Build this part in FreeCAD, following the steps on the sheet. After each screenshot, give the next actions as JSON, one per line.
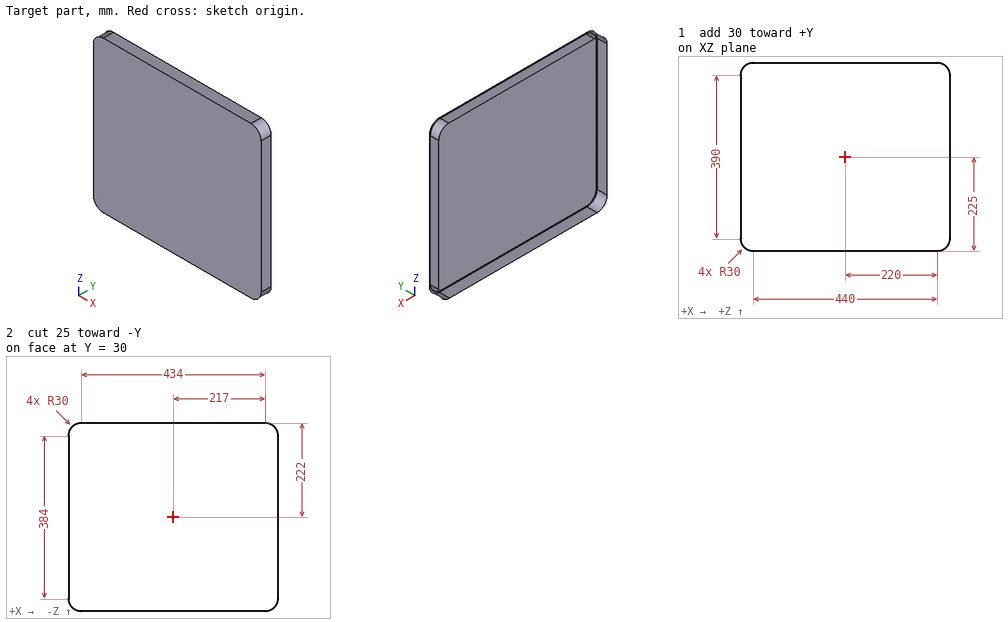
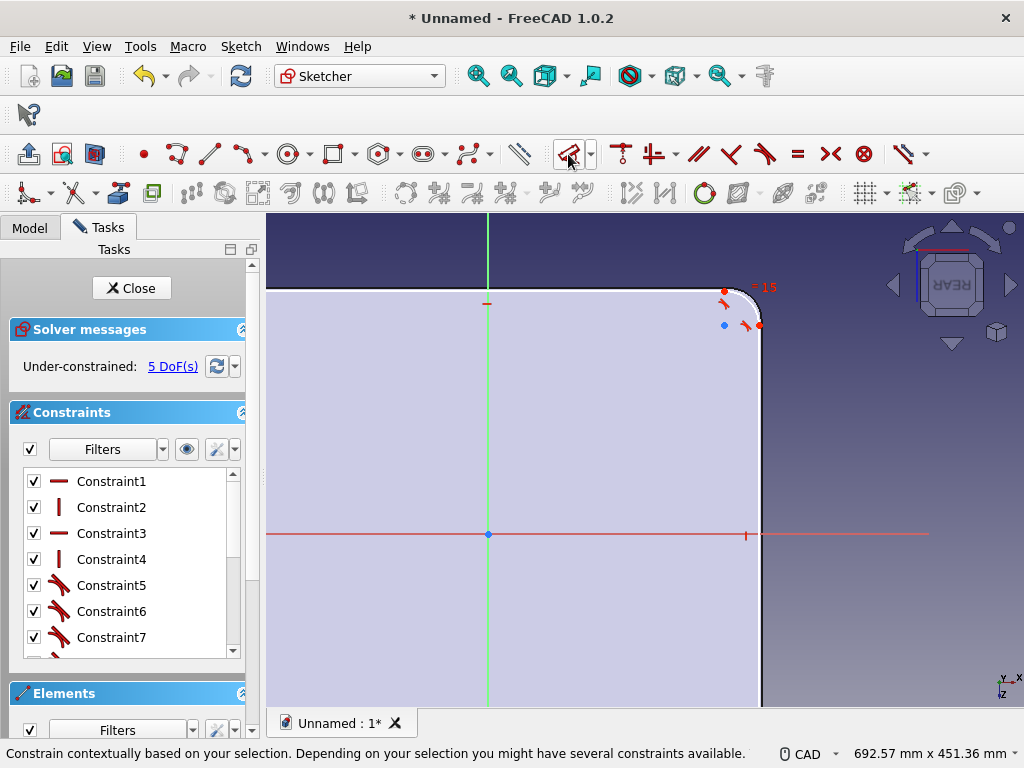
{"action": "scroll", "coordinate": [756, 309], "scroll_direction": "down", "scroll_amount": 2}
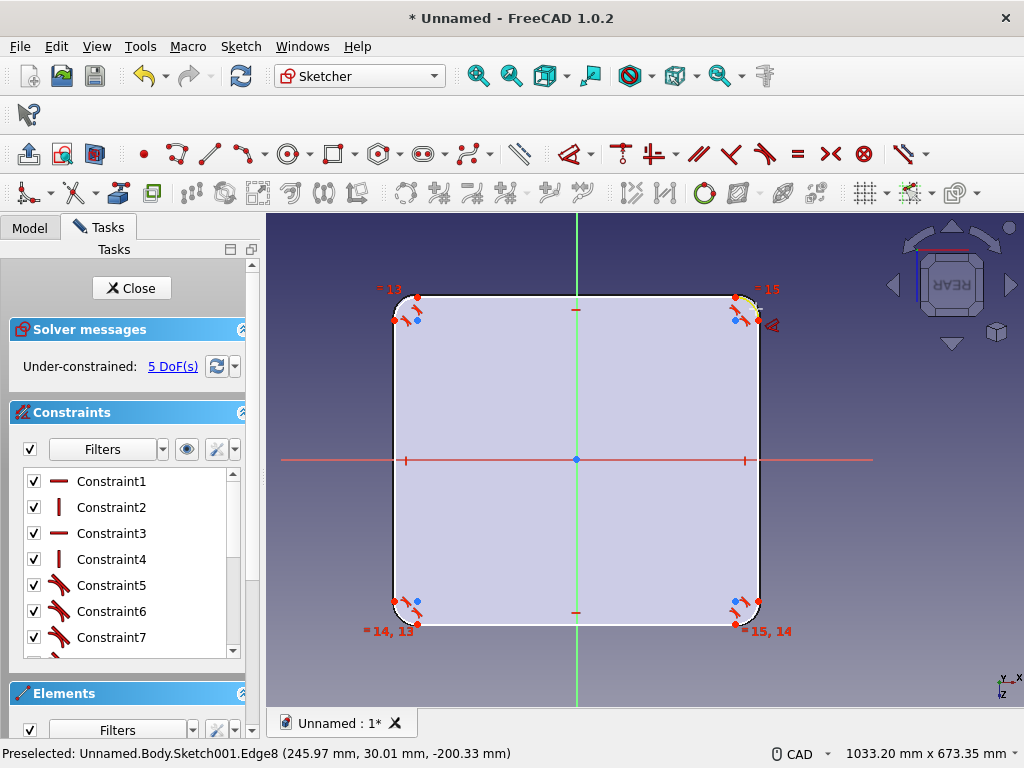
{"action": "scroll", "coordinate": [407, 300], "scroll_direction": "up", "scroll_amount": 3}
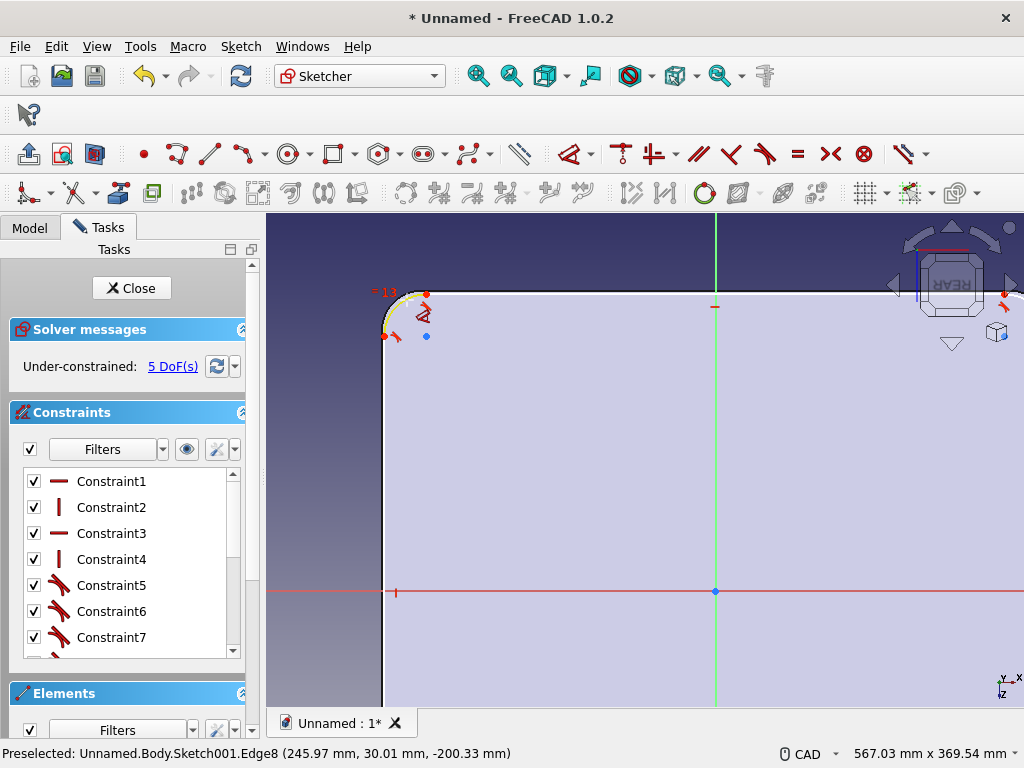
{"action": "left_click", "coordinate": [407, 299]}
{"action": "left_click", "coordinate": [392, 271]}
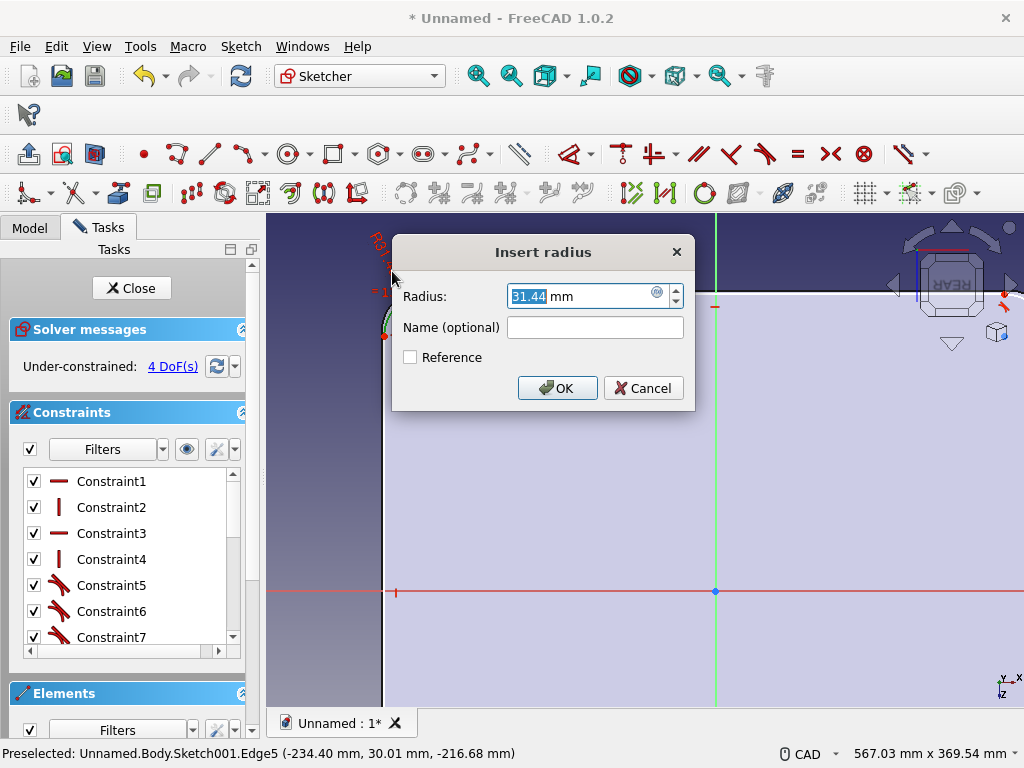
{"action": "type", "text": "30"}
{"action": "key", "text": "Return"}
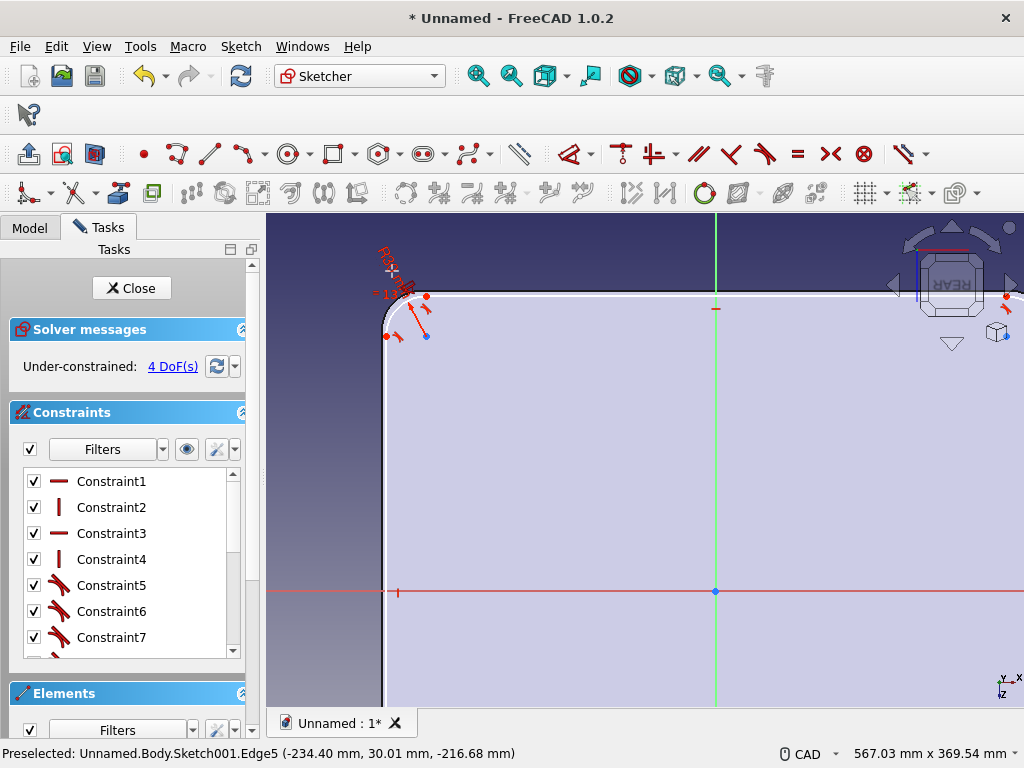
{"action": "left_click", "coordinate": [832, 296]}
{"action": "left_click", "coordinate": [643, 262]}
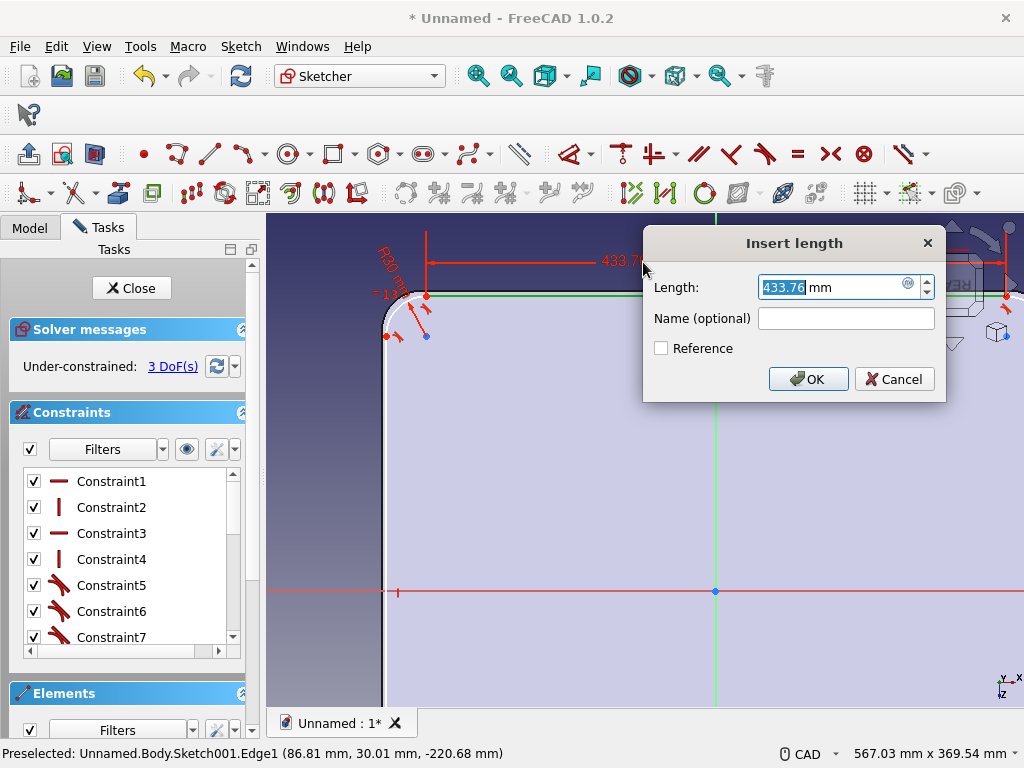
{"action": "type", "text": "434"}
{"action": "key", "text": "Return"}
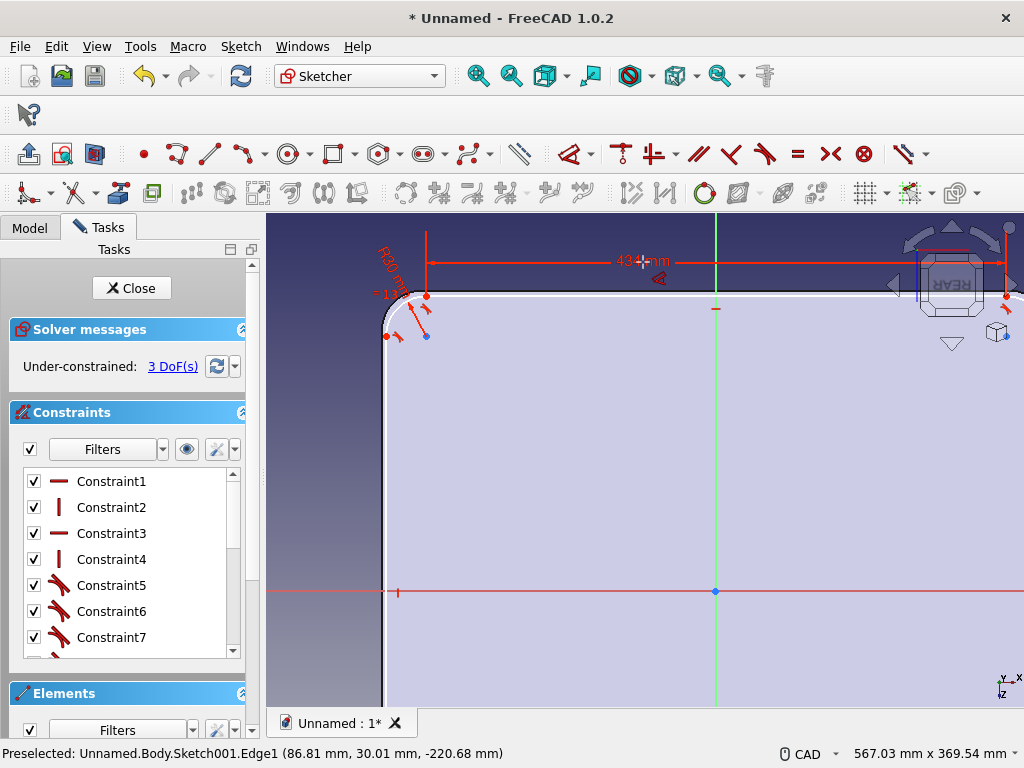
{"action": "left_click", "coordinate": [386, 490]}
{"action": "left_click", "coordinate": [352, 508]}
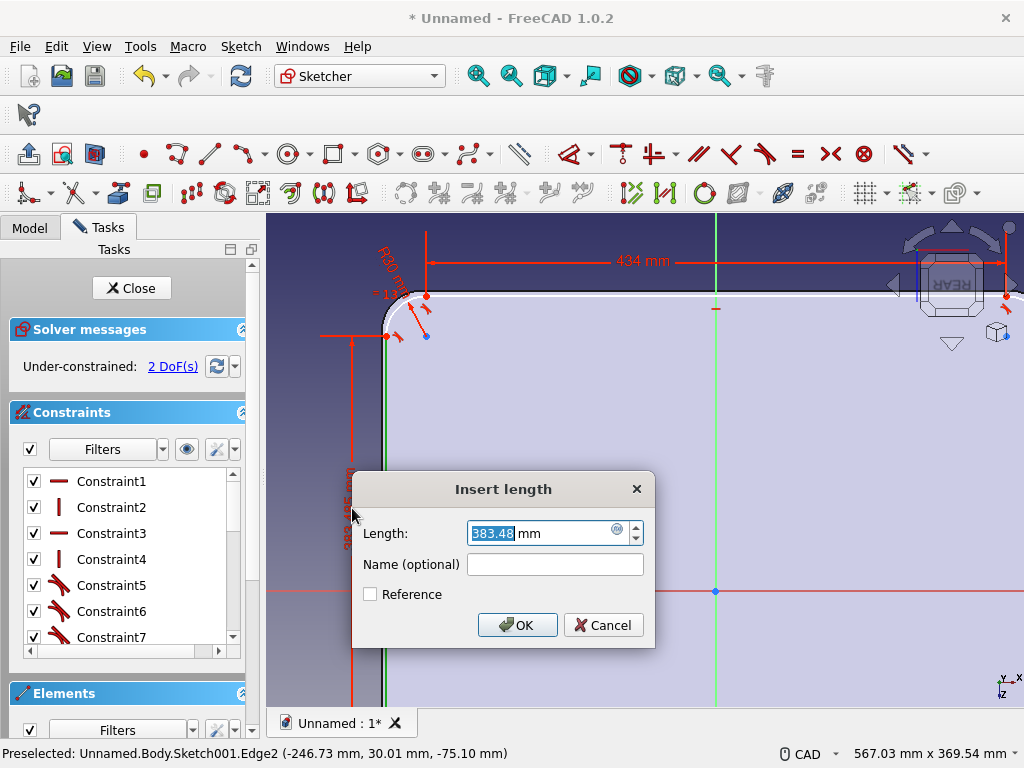
{"action": "type", "text": "384"}
{"action": "key", "text": "Return"}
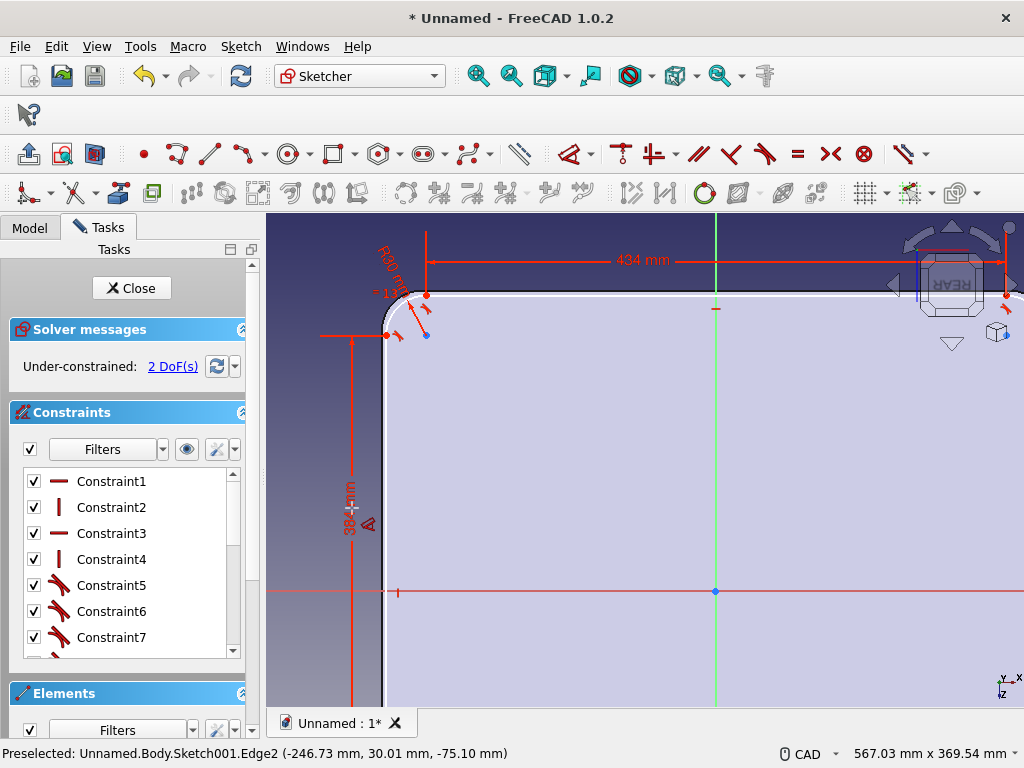
{"action": "scroll", "coordinate": [407, 300], "scroll_direction": "down", "scroll_amount": 3}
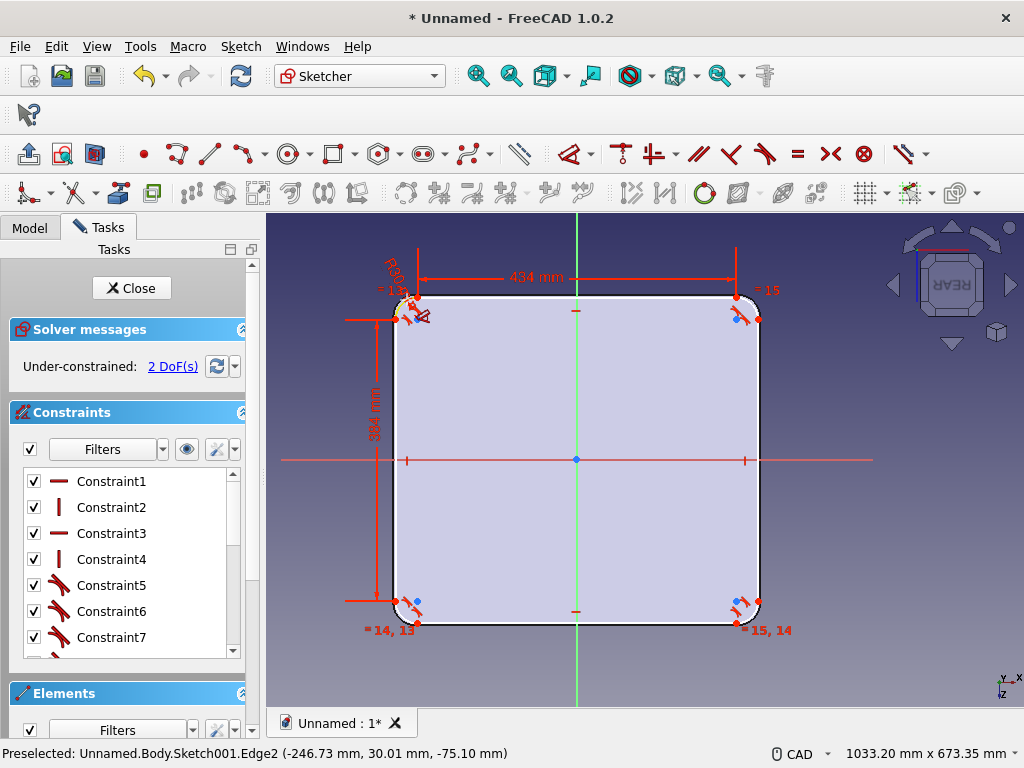
{"action": "left_click", "coordinate": [736, 298]}
{"action": "left_click", "coordinate": [656, 264]}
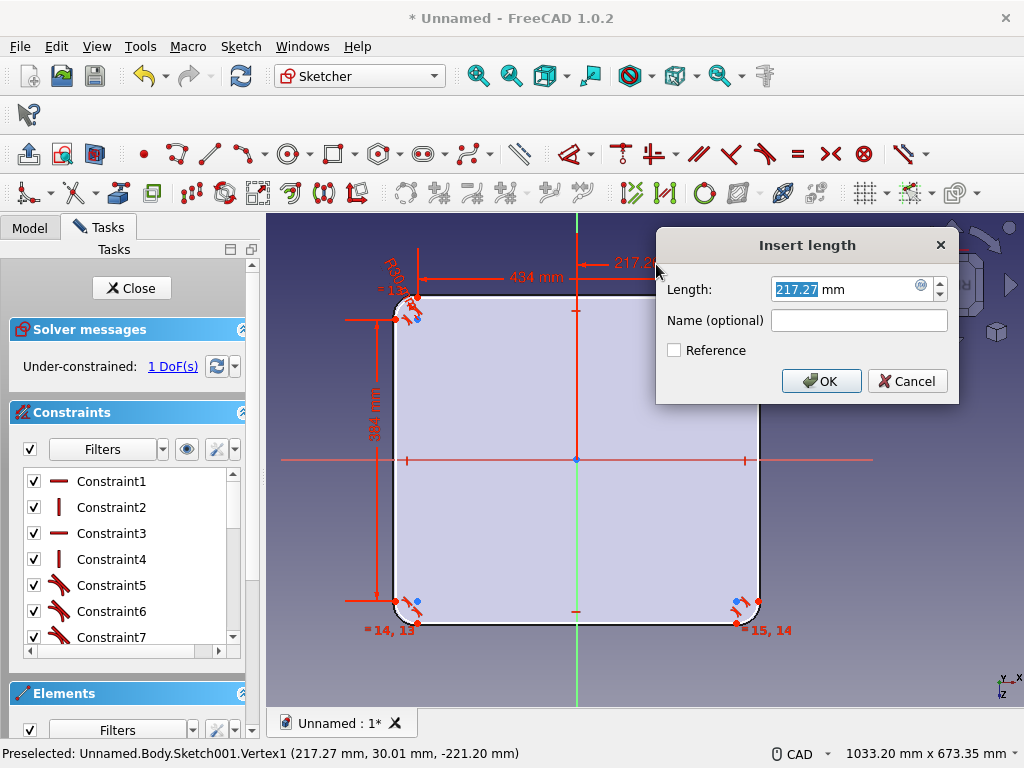
{"action": "type", "text": "217"}
{"action": "key", "text": "Return"}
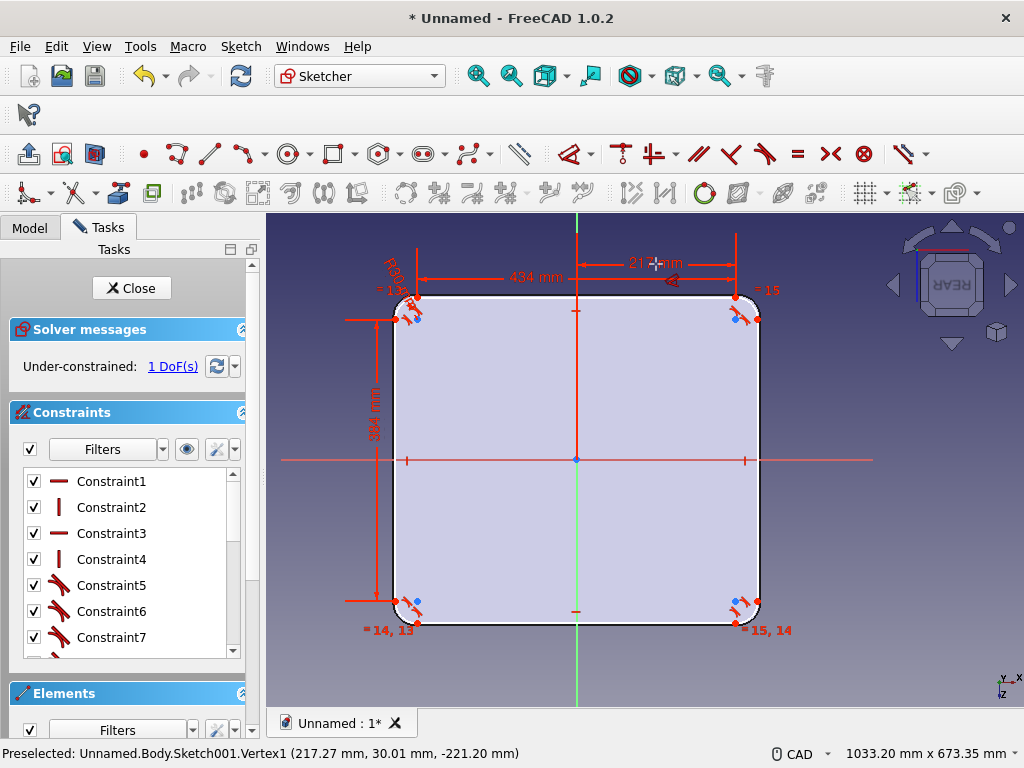
{"action": "left_click", "coordinate": [736, 298]}
{"action": "left_click", "coordinate": [543, 379]}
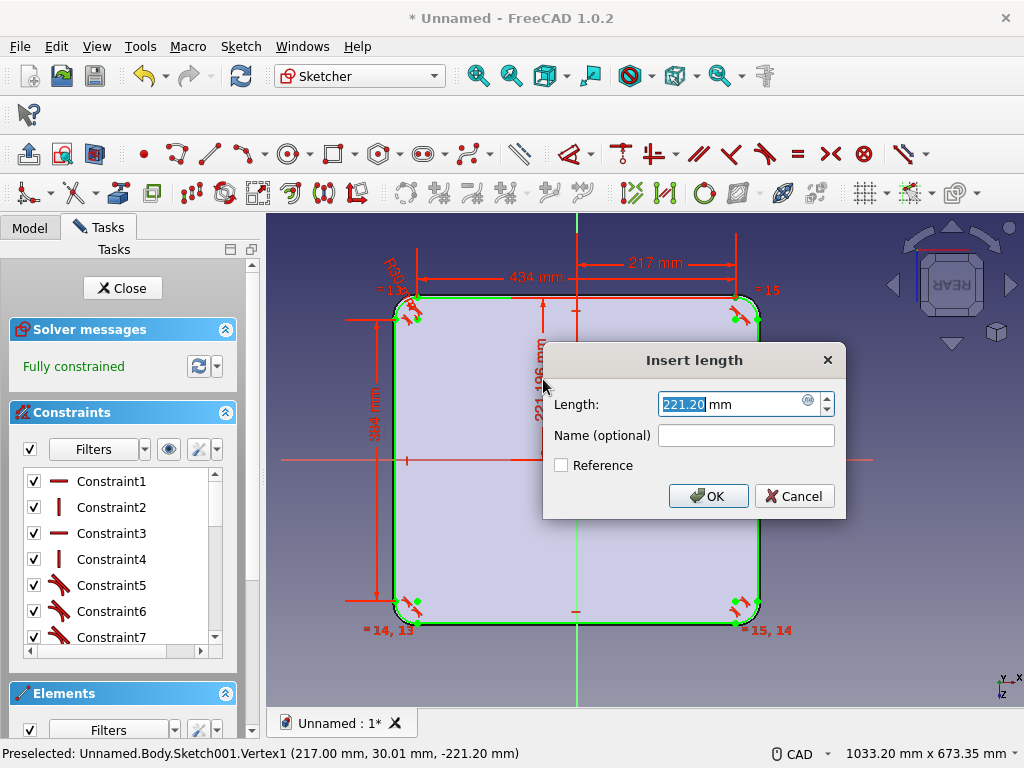
{"action": "type", "text": "222"}
{"action": "key", "text": "Return"}
{"action": "key", "text": "Escape"}